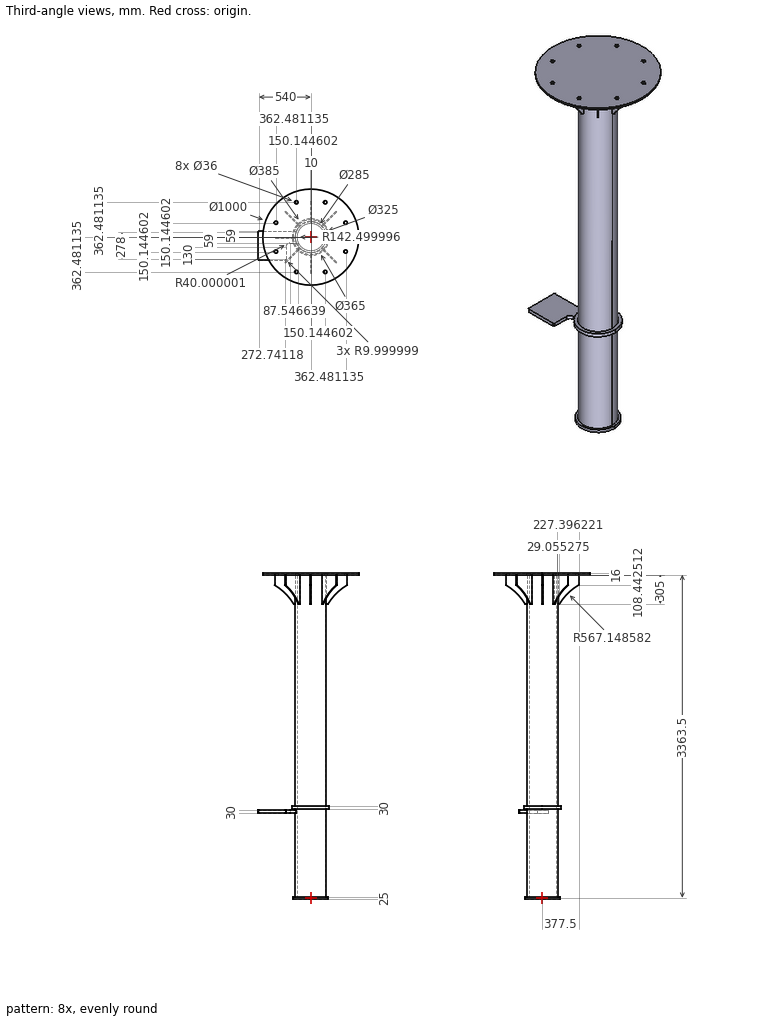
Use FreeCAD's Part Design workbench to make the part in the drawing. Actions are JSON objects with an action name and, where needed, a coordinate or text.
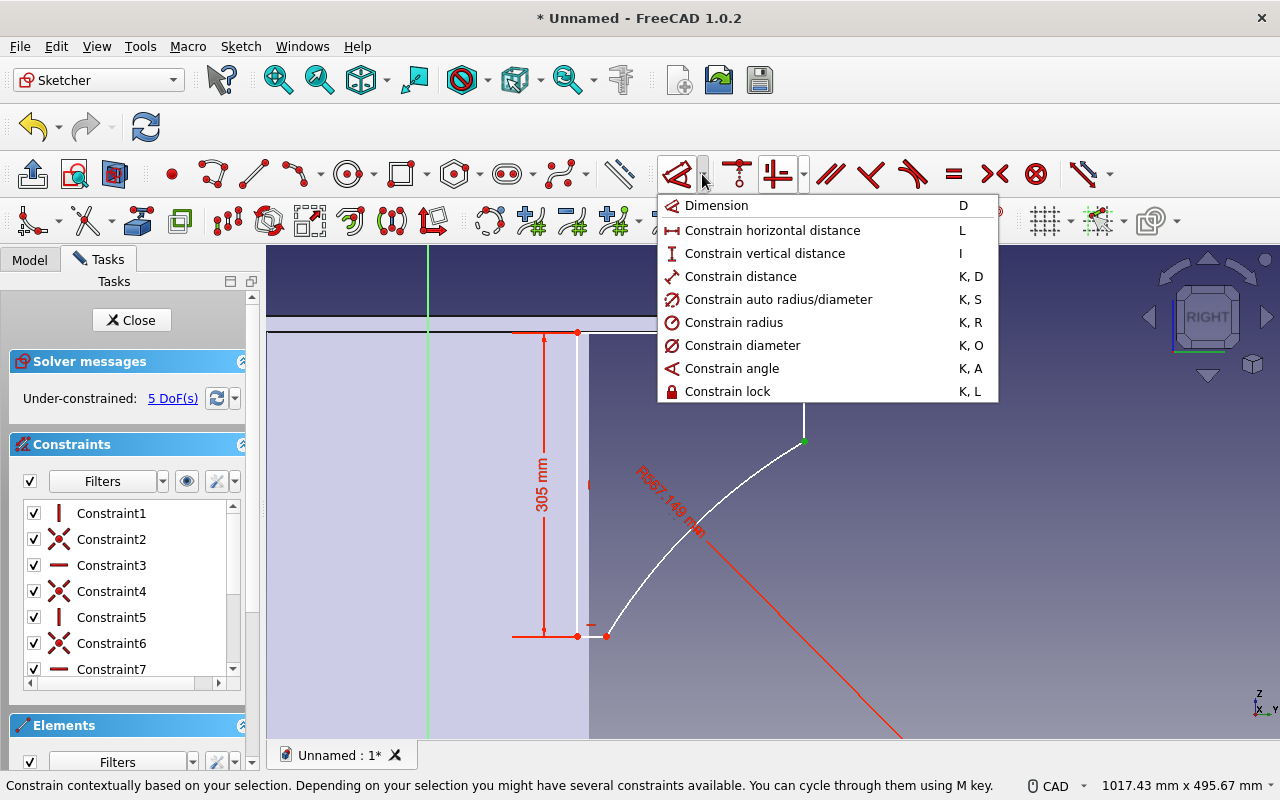
{"action": "left_click", "coordinate": [828, 230]}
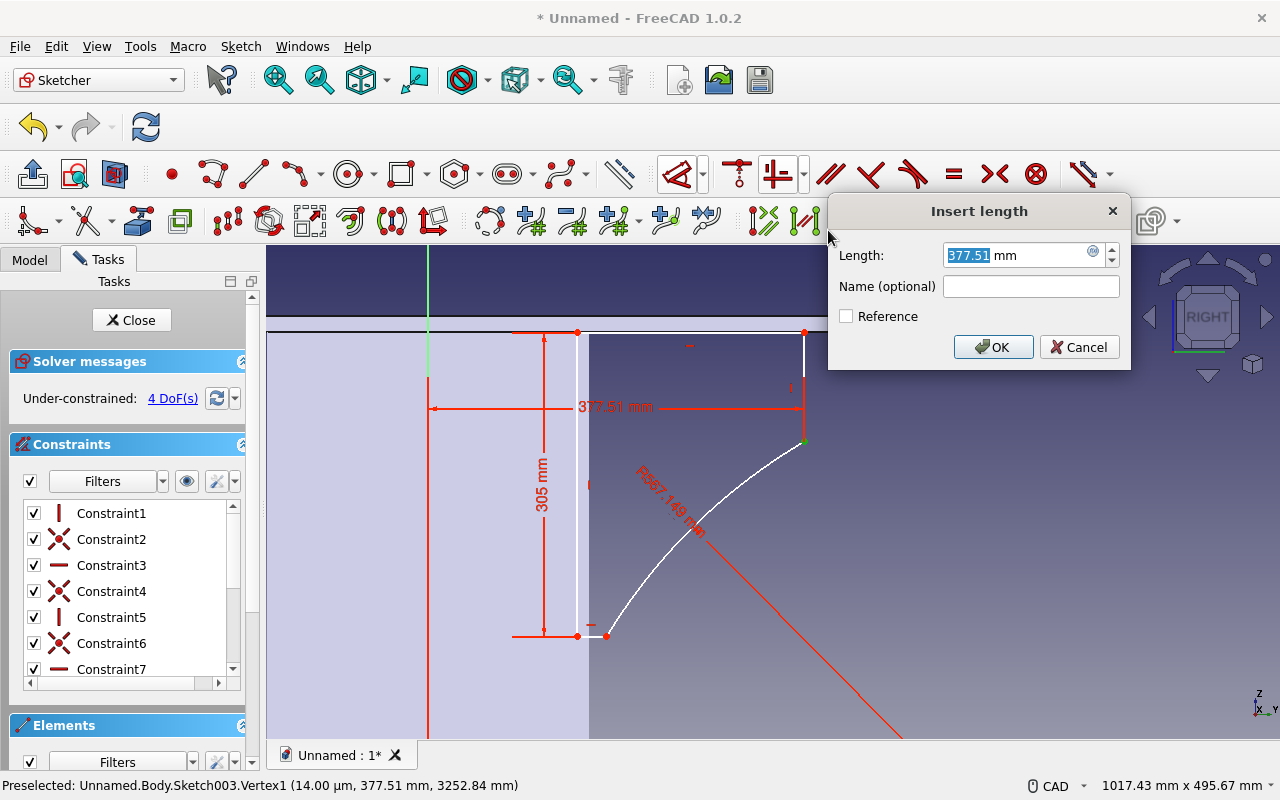
{"action": "type", "text": "377.5"}
{"action": "key", "text": "Return"}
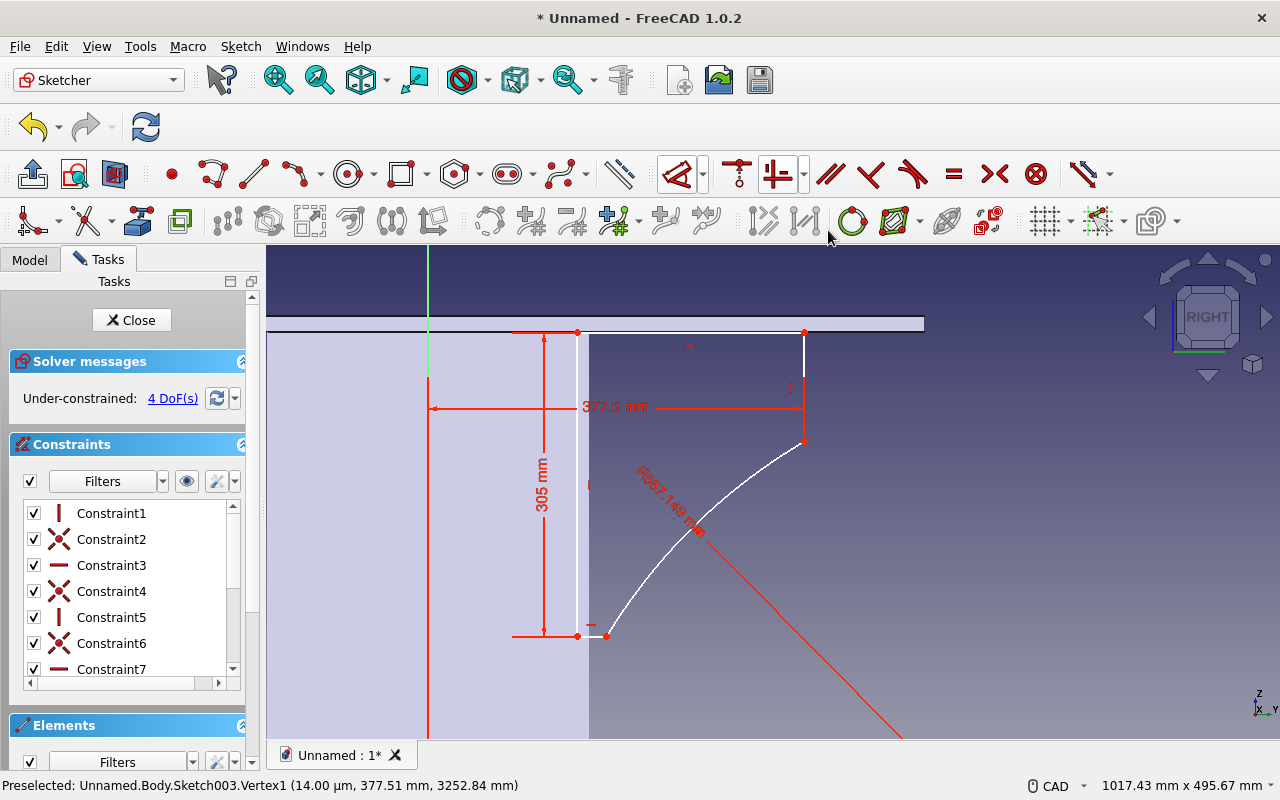
{"action": "left_click", "coordinate": [804, 333]}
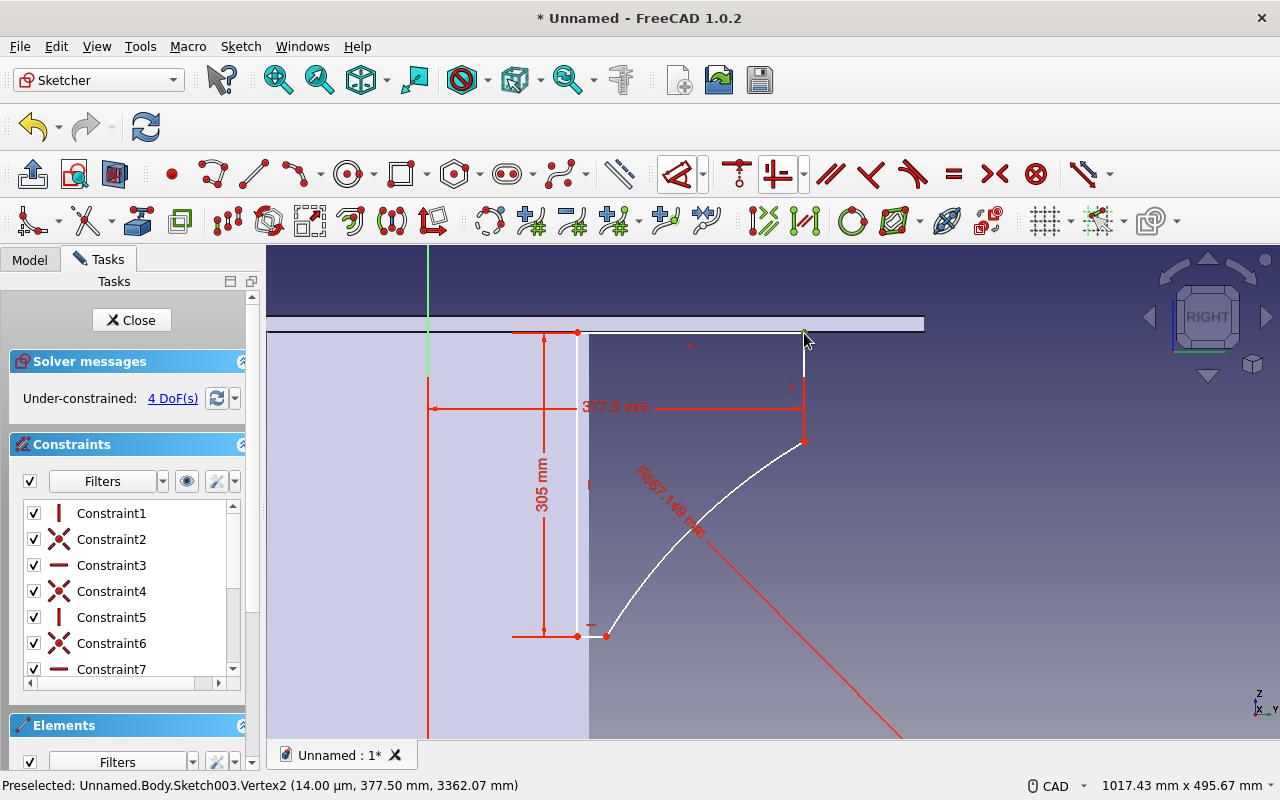
{"action": "key", "text": "i"}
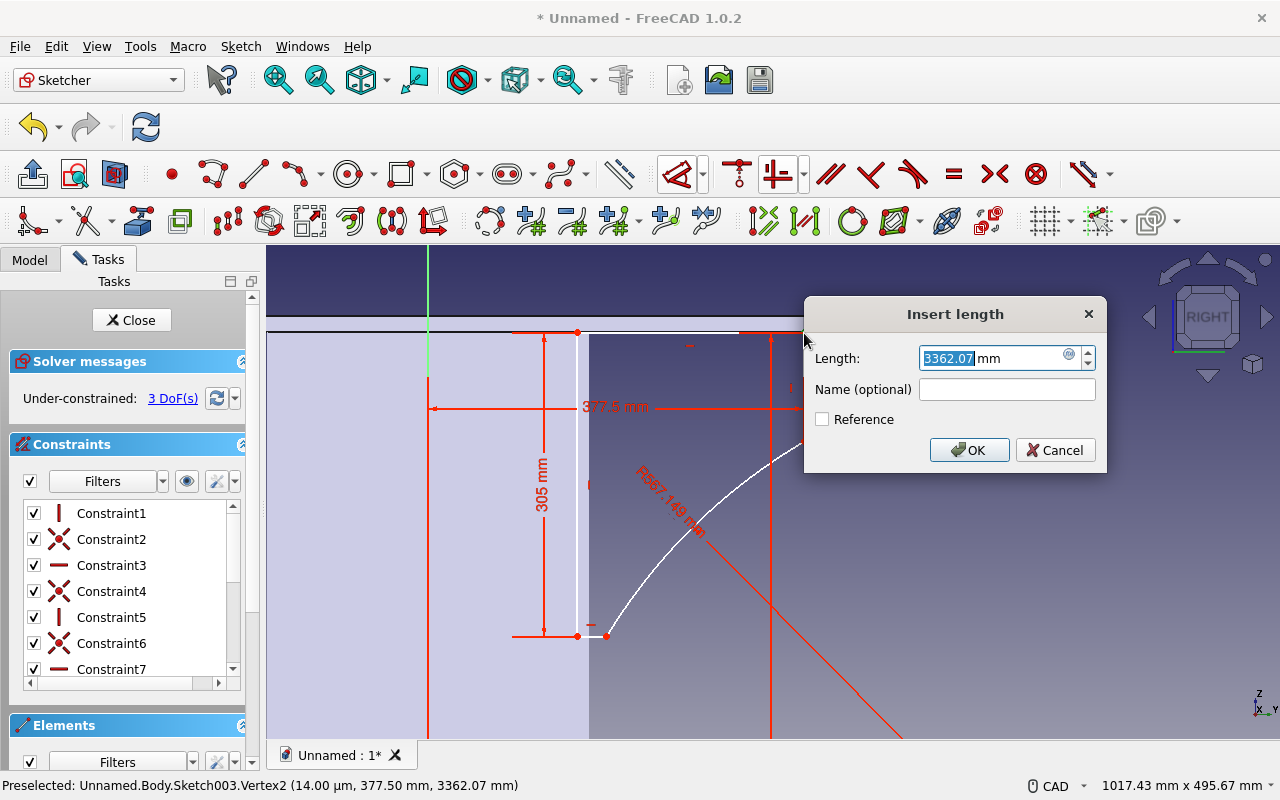
{"action": "type", "text": "3363.5"}
{"action": "key", "text": "Return"}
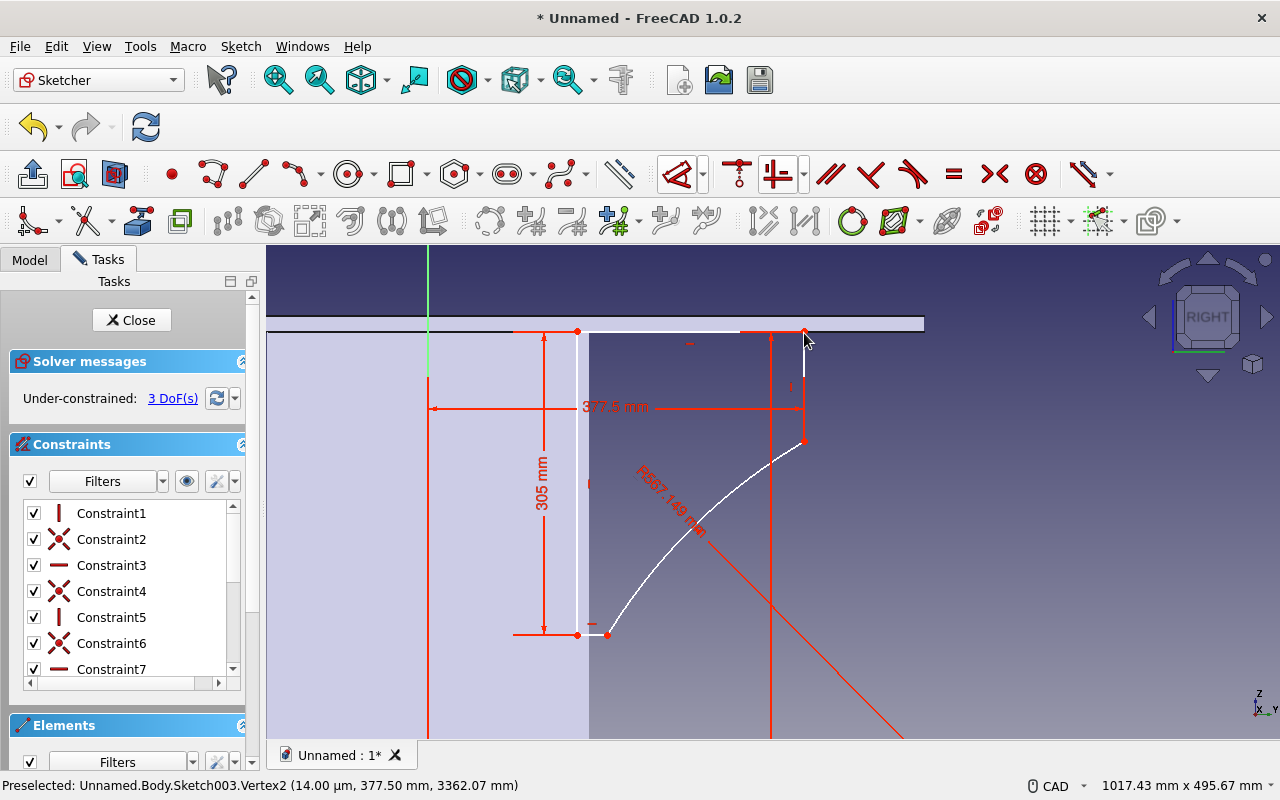
{"action": "scroll", "coordinate": [586, 635], "scroll_direction": "up", "scroll_amount": 3}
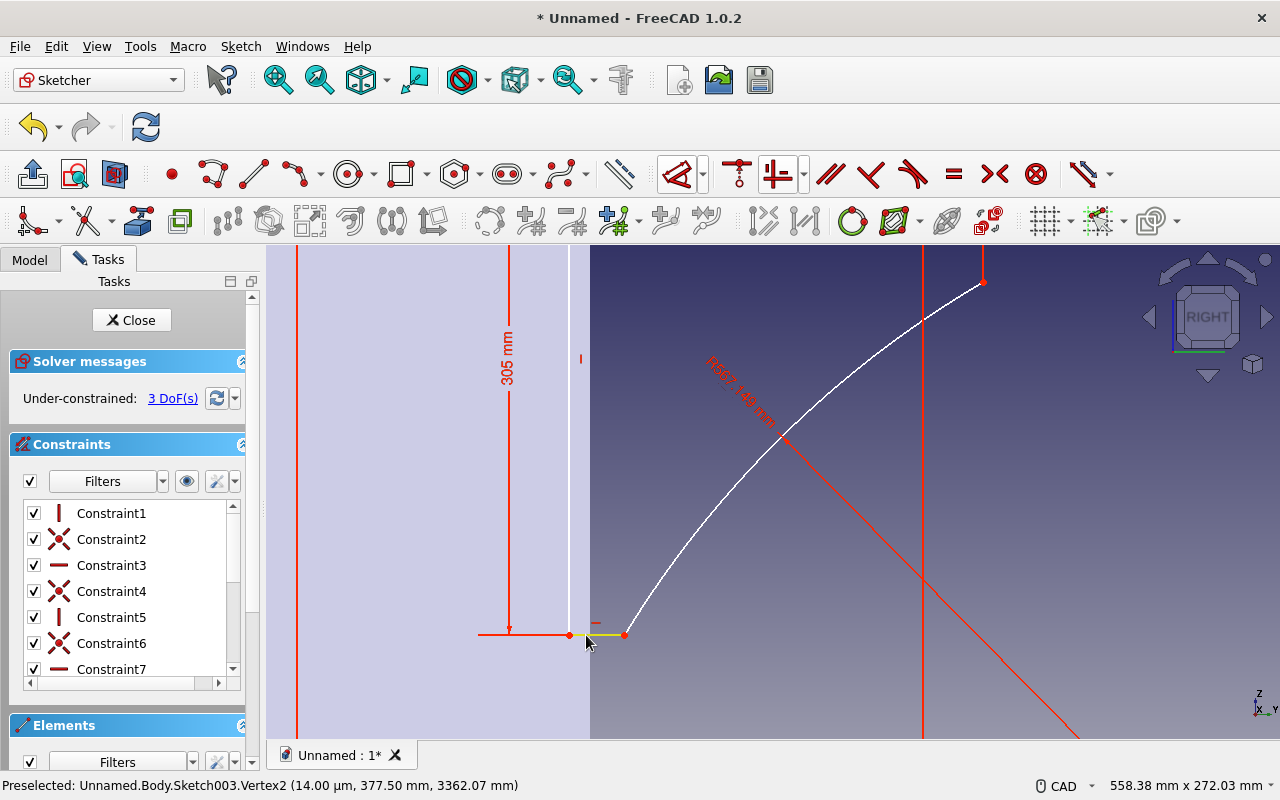
{"action": "left_click", "coordinate": [586, 635]}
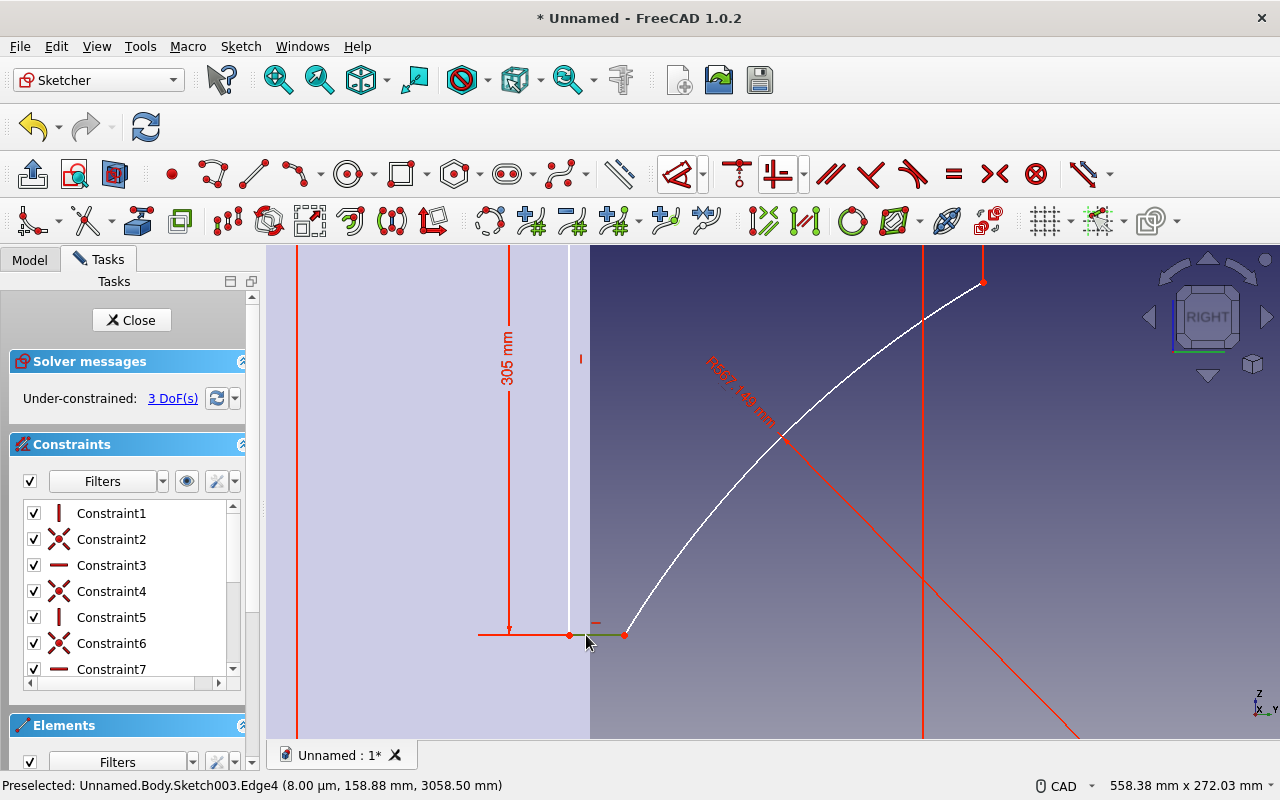
{"action": "key", "text": "l"}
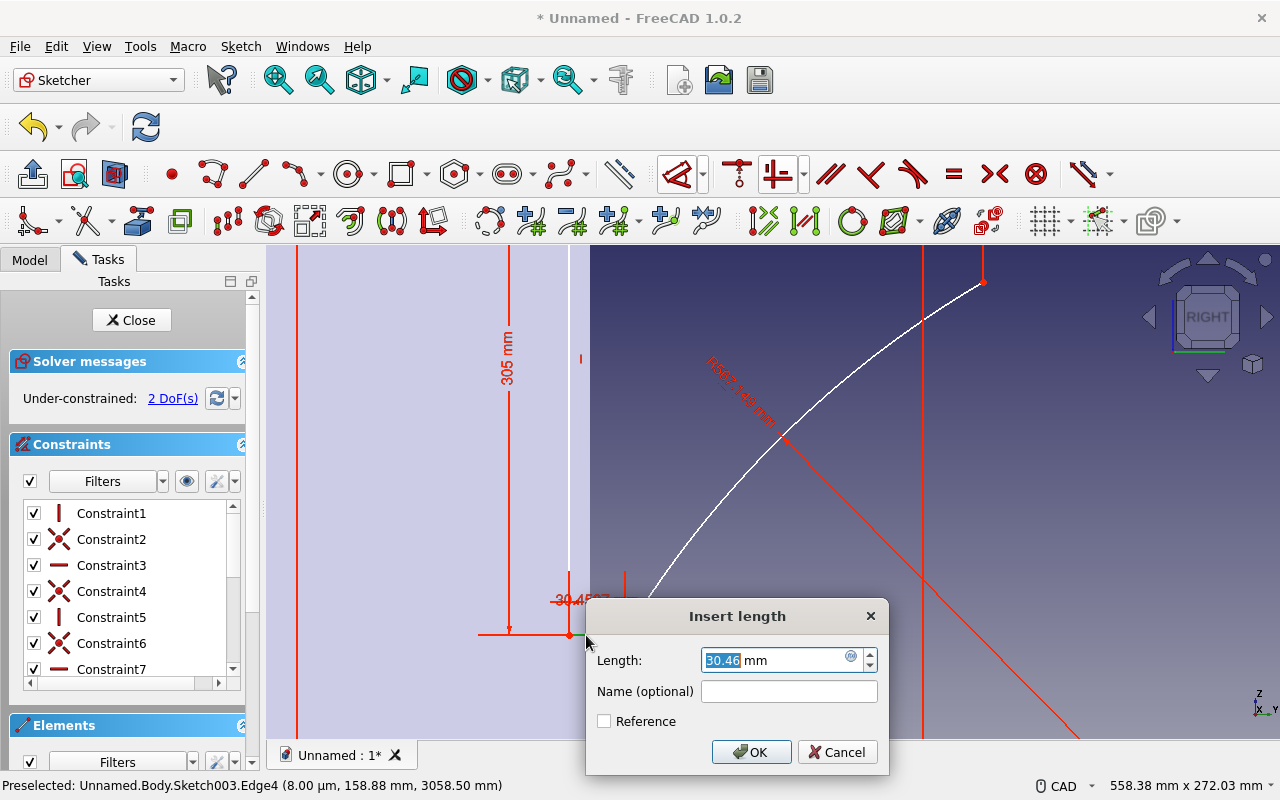
{"action": "type", "text": "29.055275"}
{"action": "key", "text": "Return"}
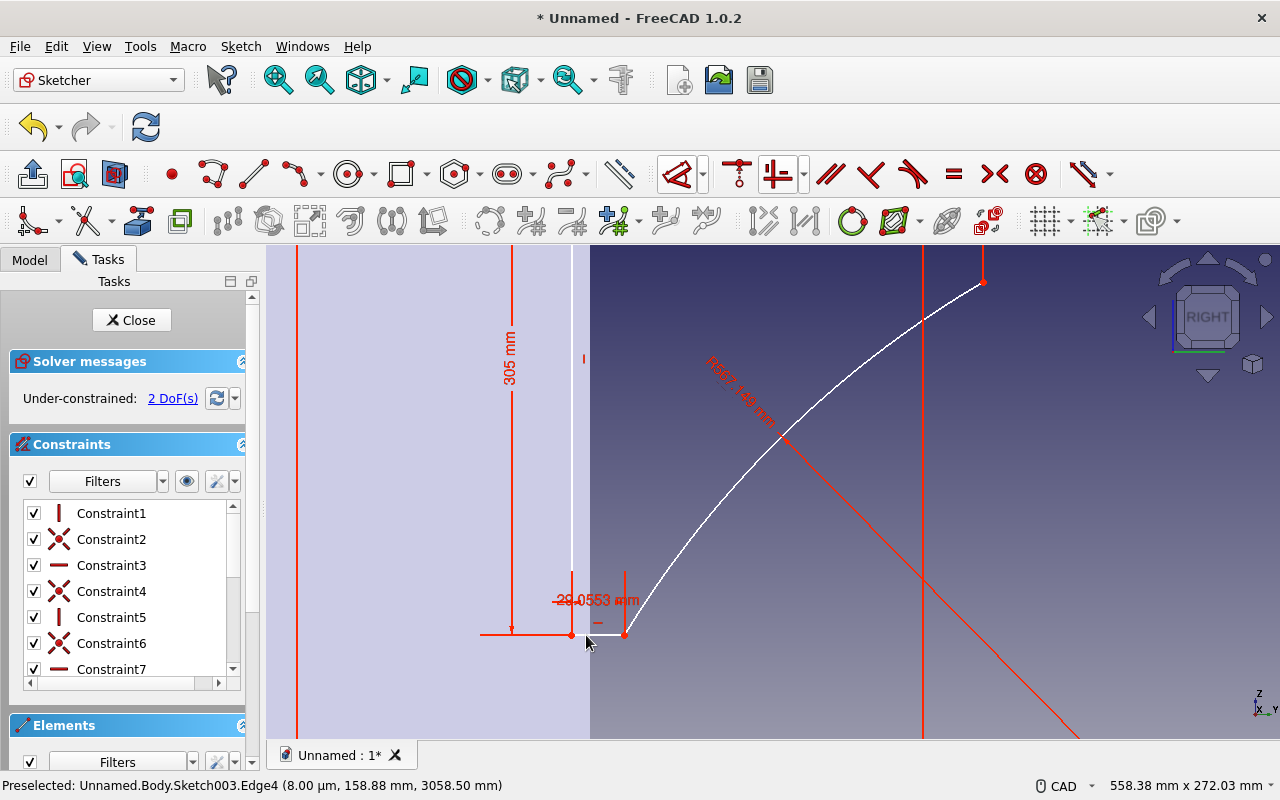
{"action": "scroll", "coordinate": [617, 655], "scroll_direction": "down", "scroll_amount": 3}